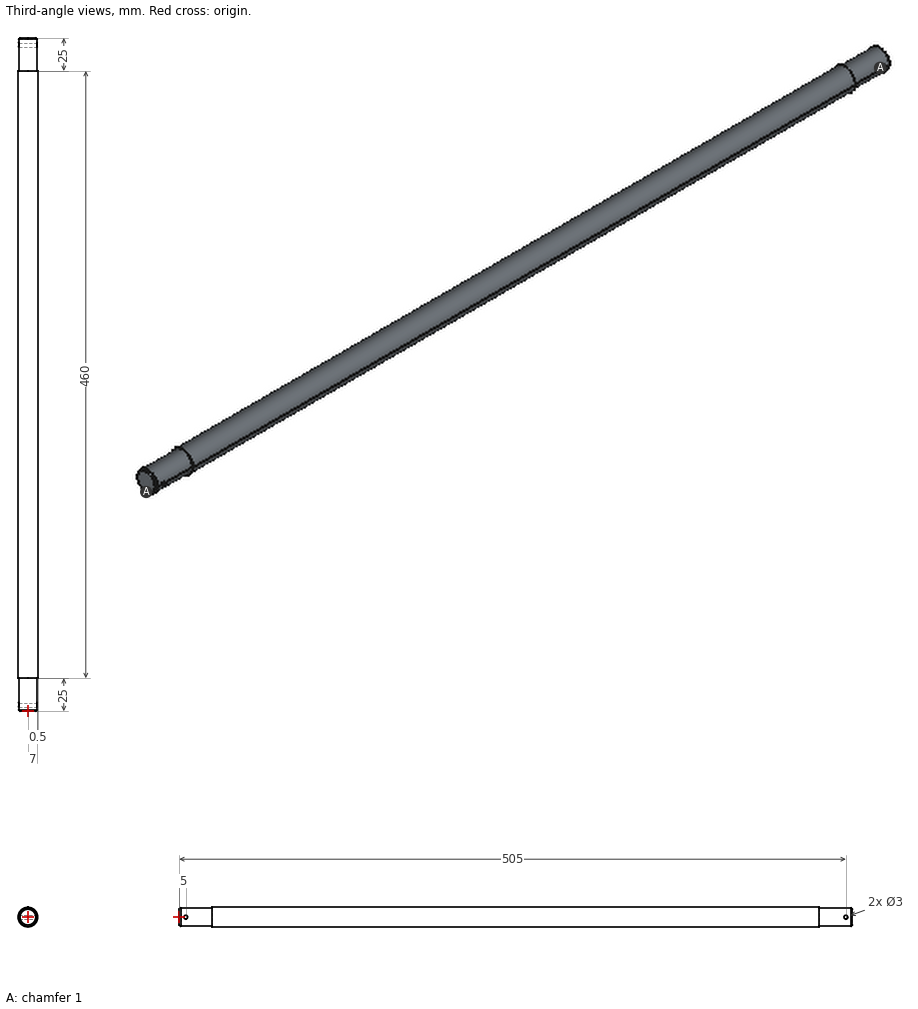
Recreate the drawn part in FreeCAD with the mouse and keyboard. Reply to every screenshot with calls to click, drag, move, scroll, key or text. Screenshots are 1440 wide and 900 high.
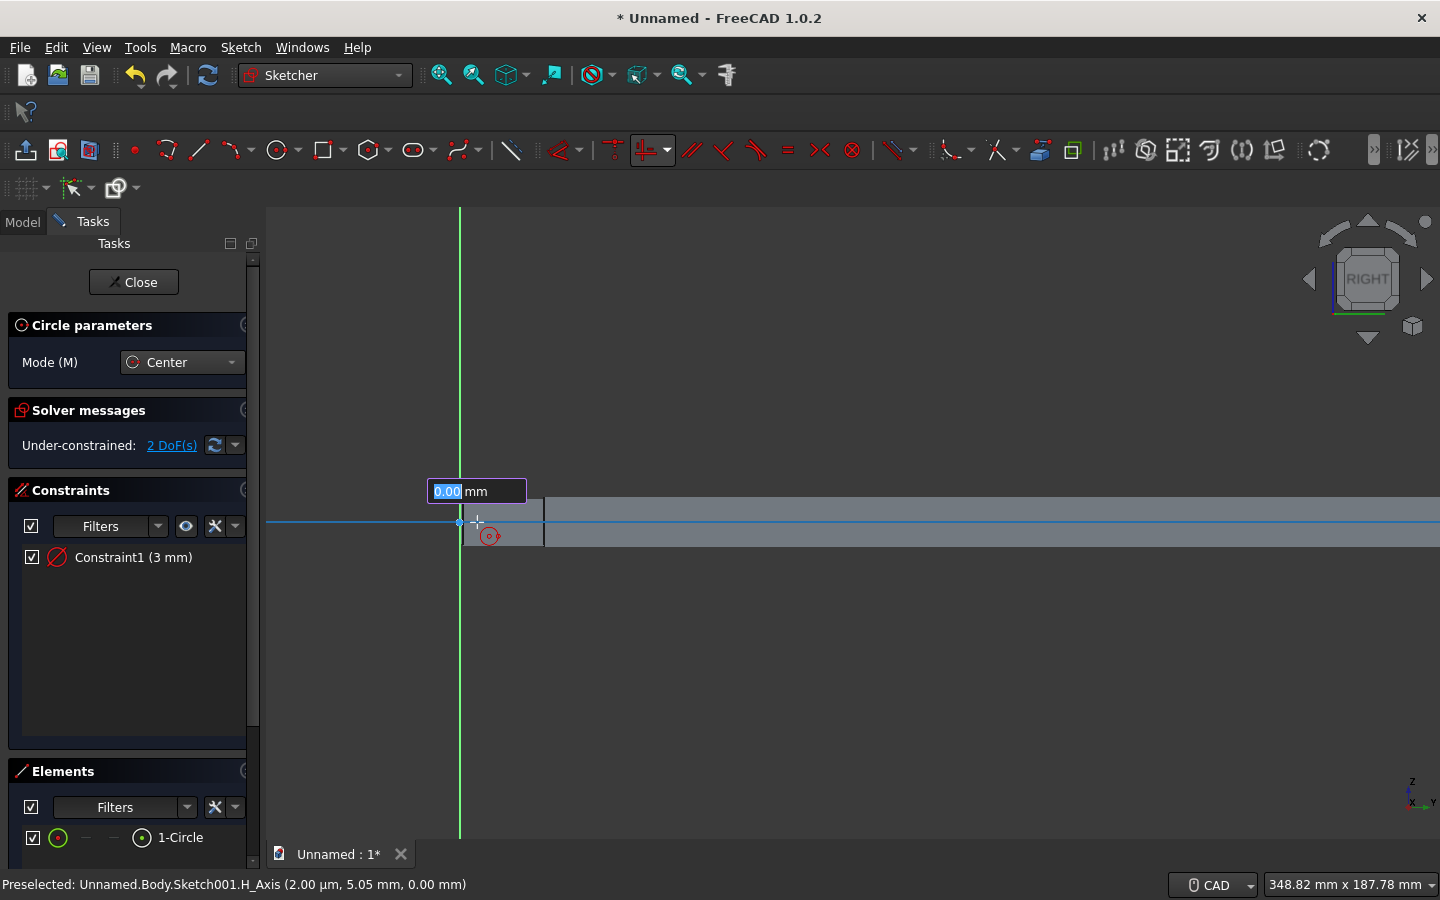
scroll(475, 527, up, 7)
move(475, 525)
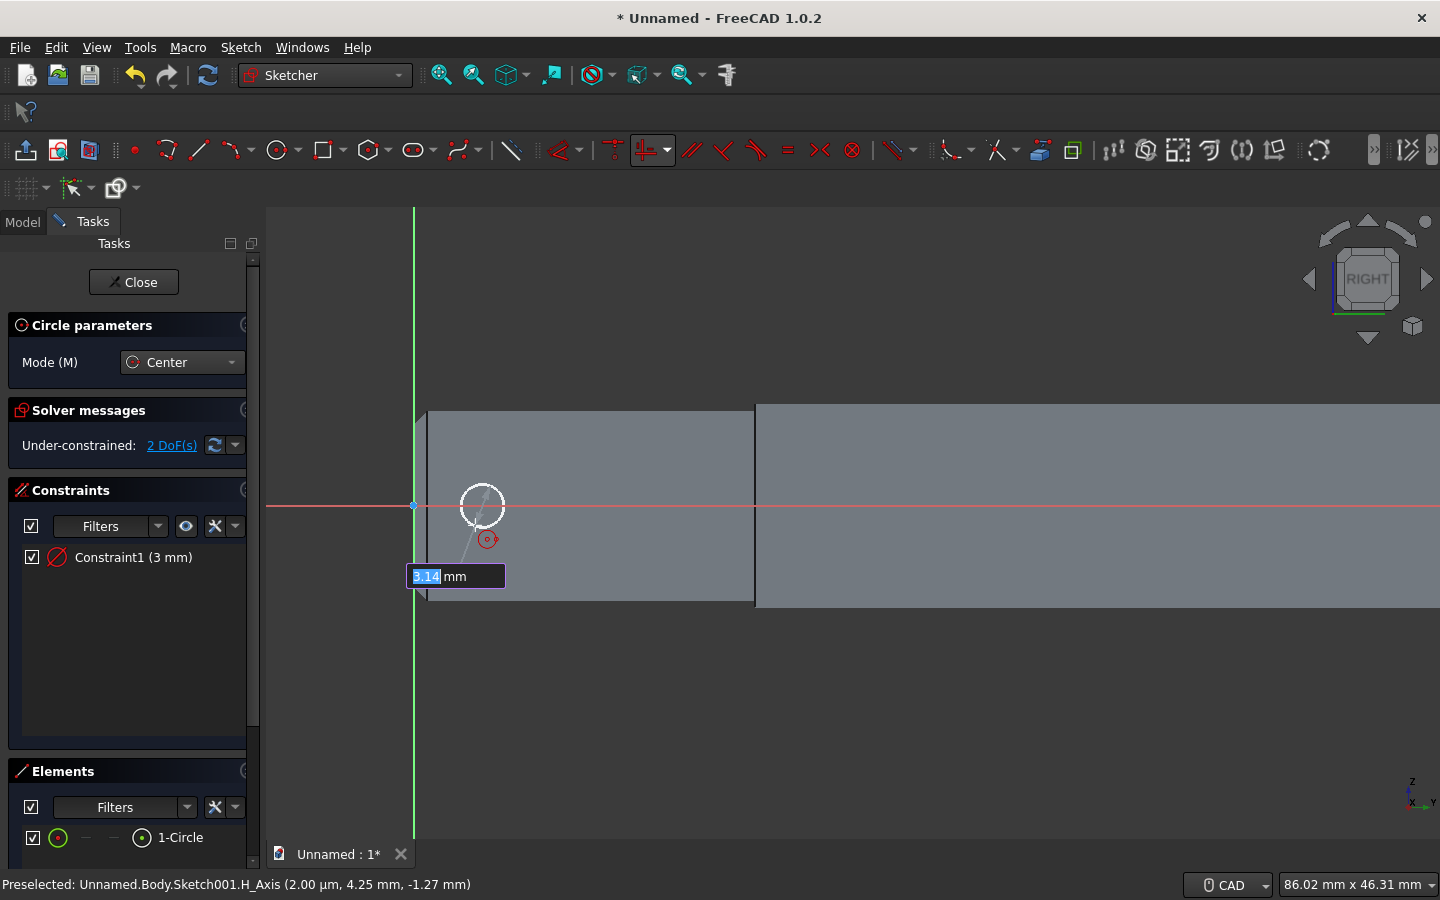
text(3)
key(Return)
key(Escape)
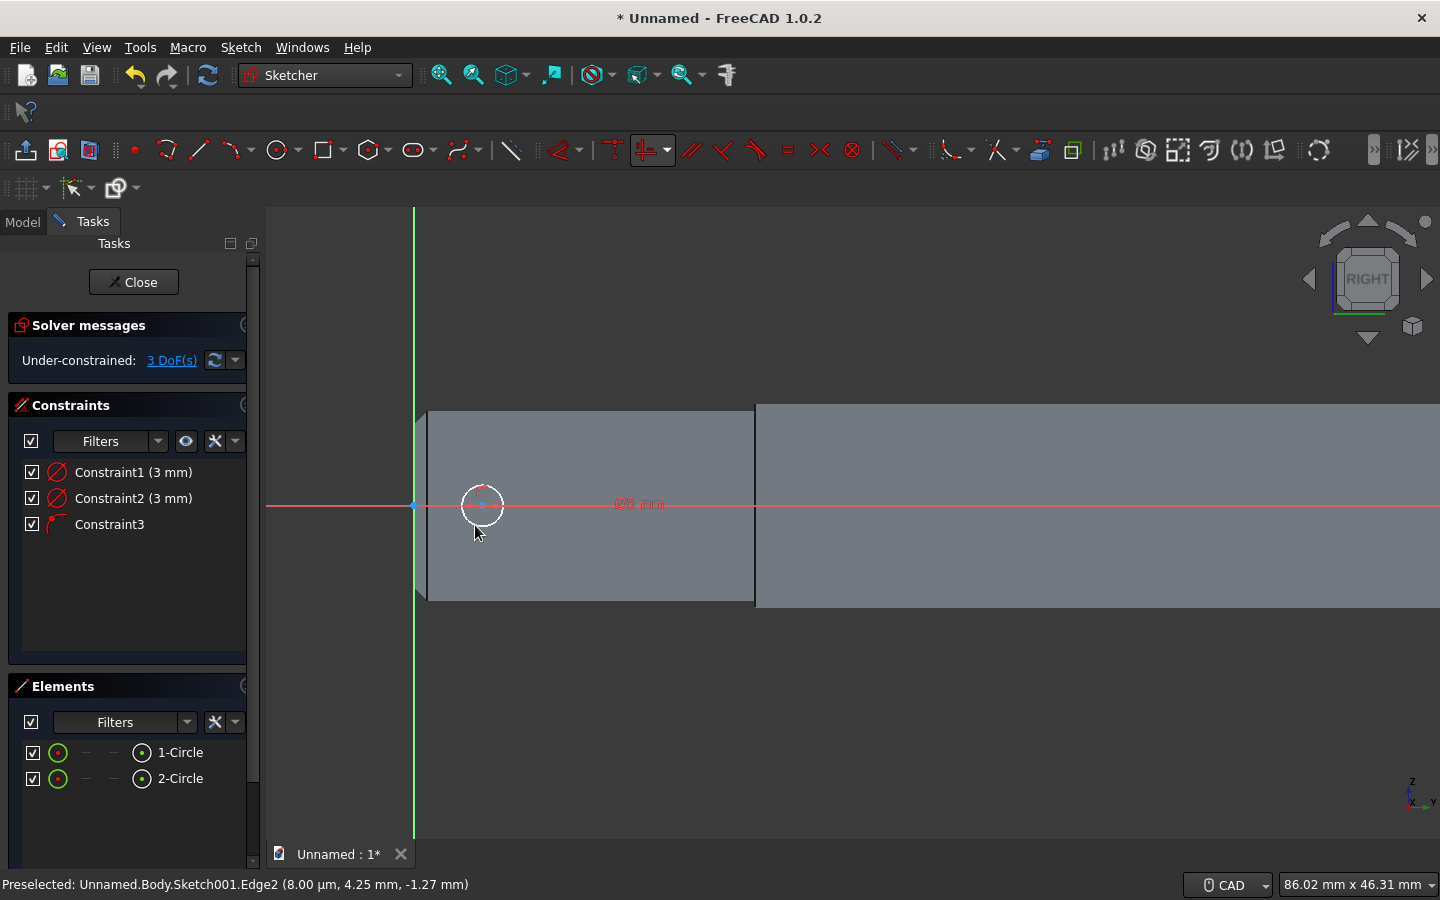
scroll(477, 525, down, 12)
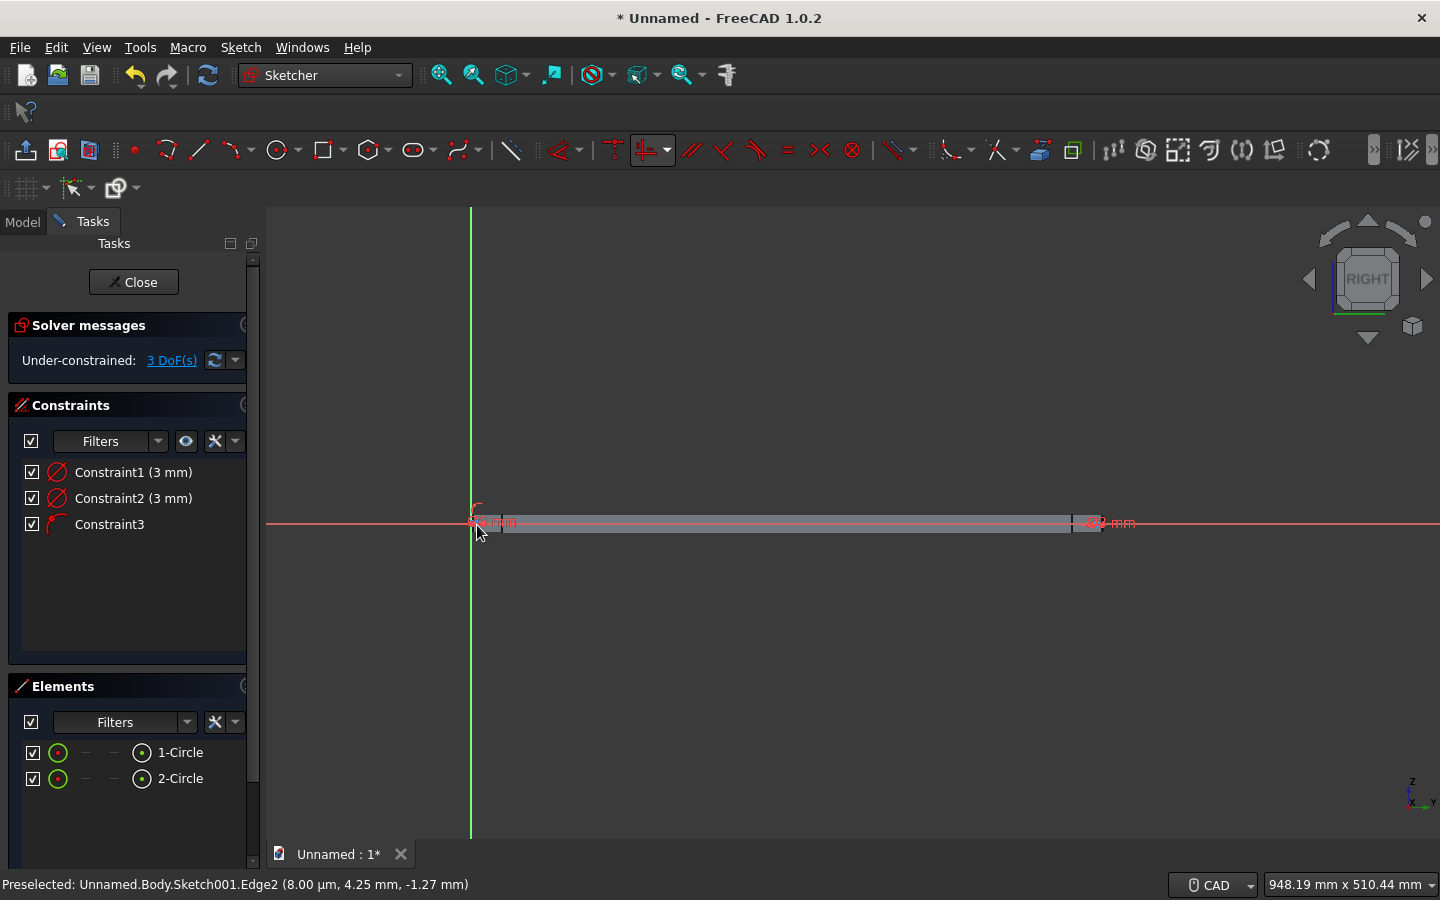
click(1097, 525)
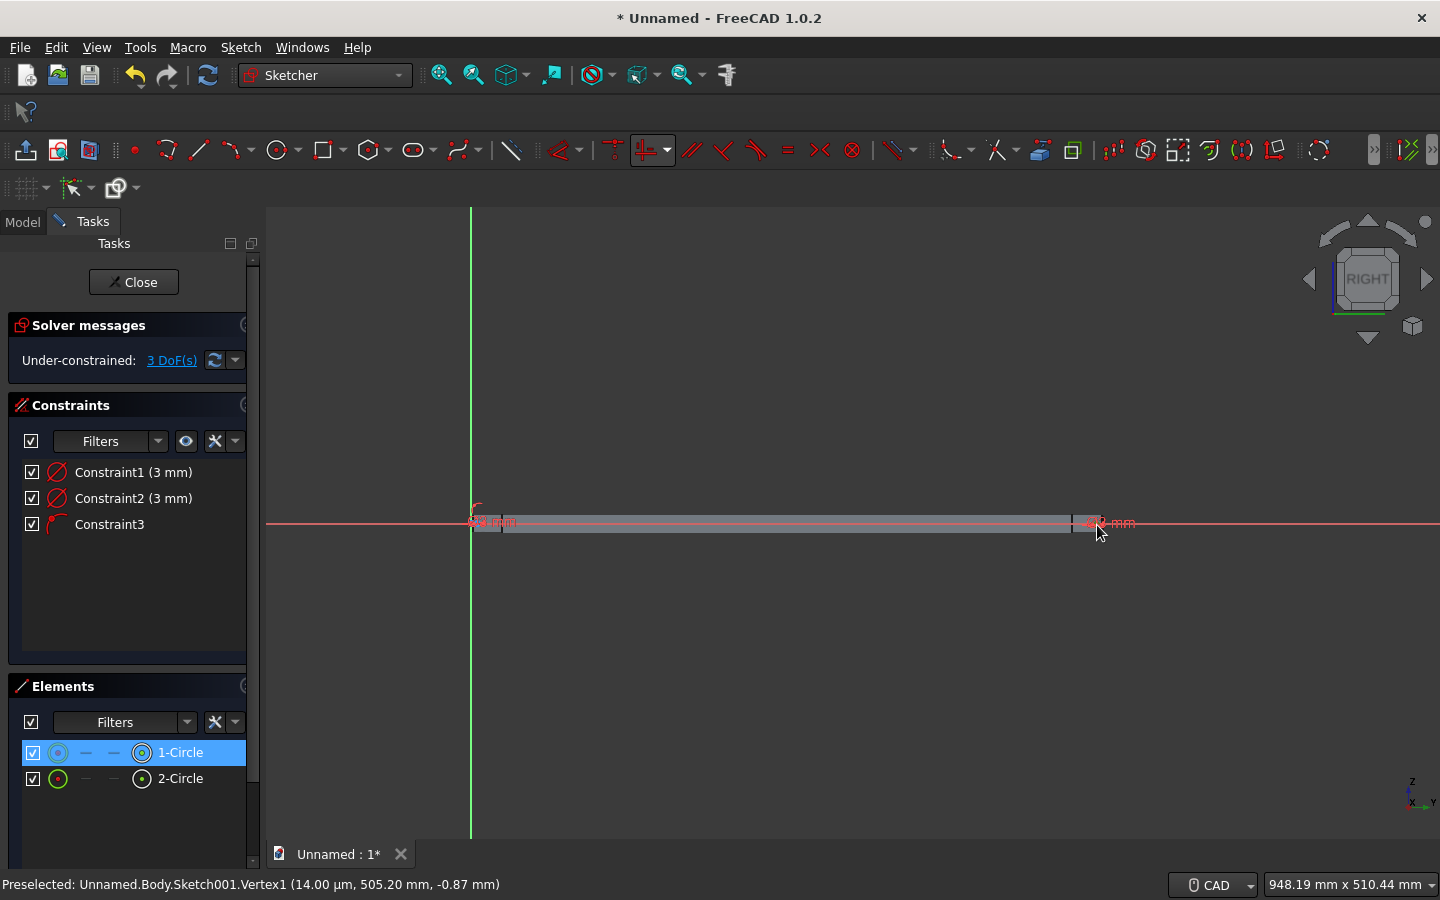
click(364, 524)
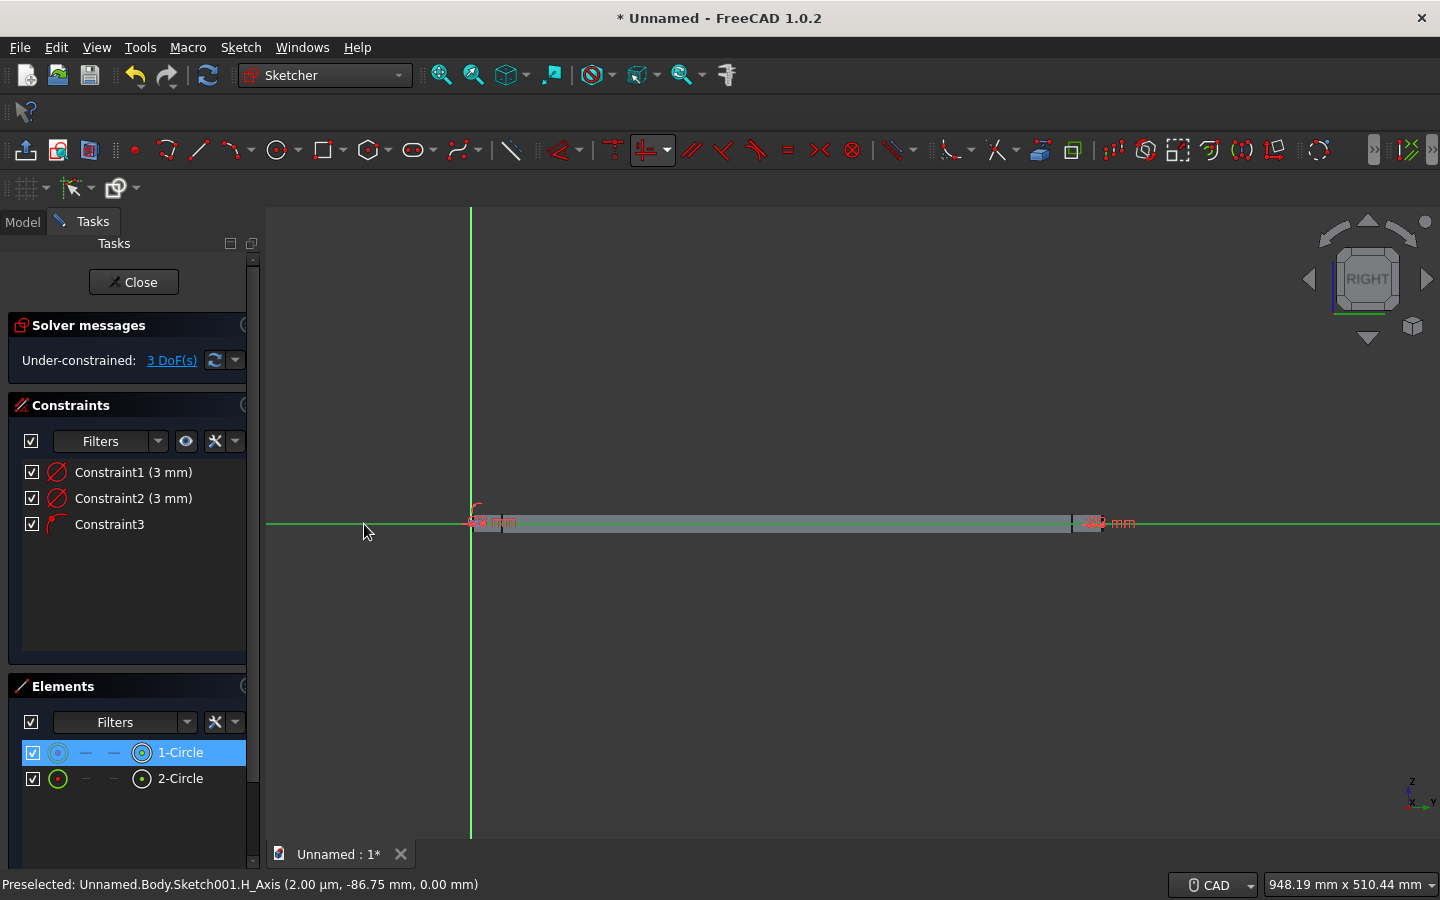
click(614, 150)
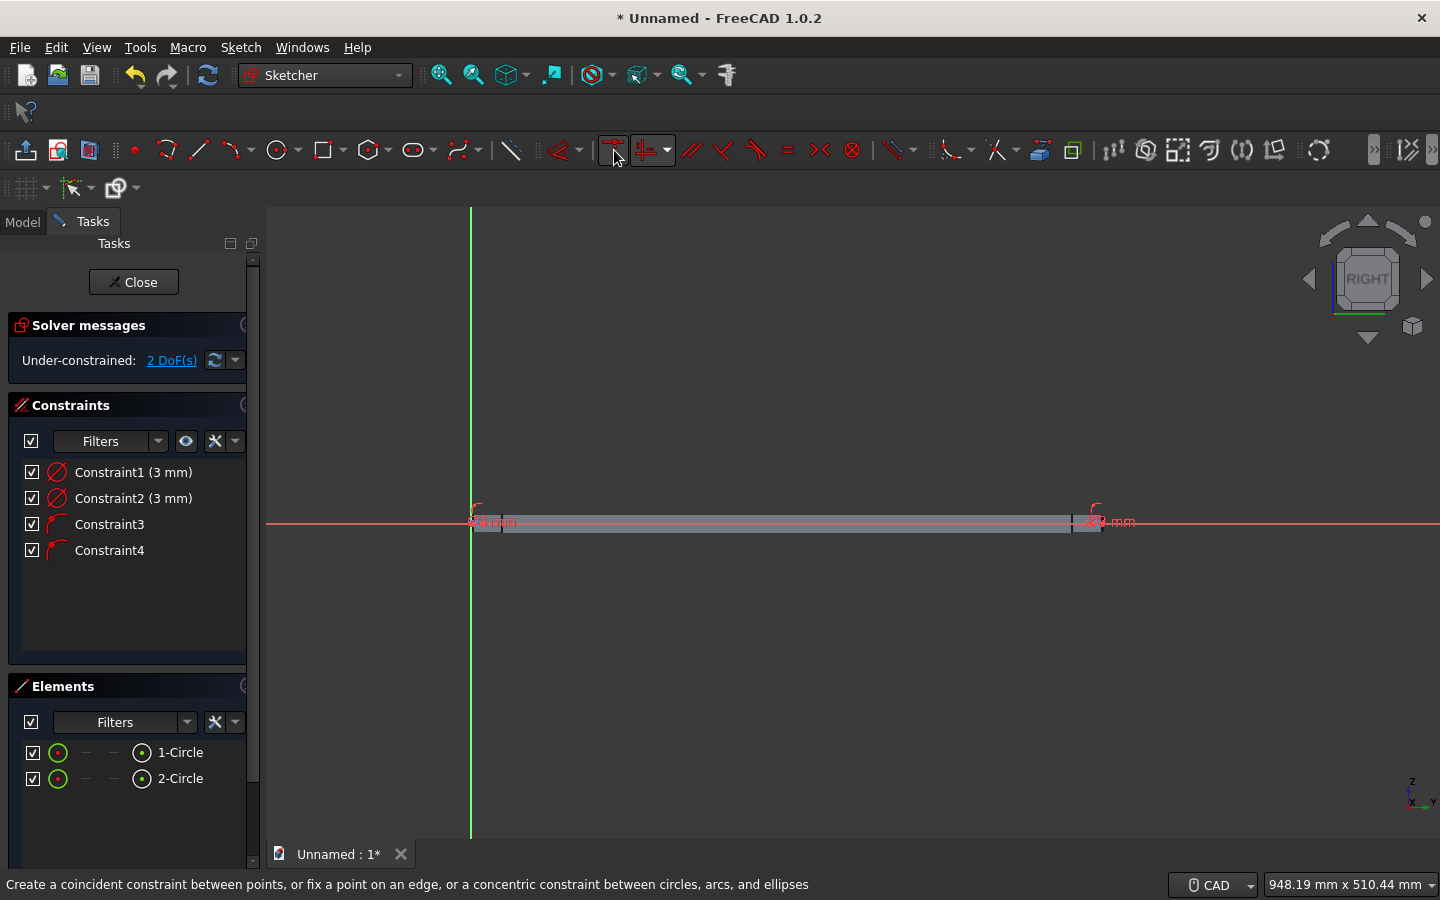
click(558, 150)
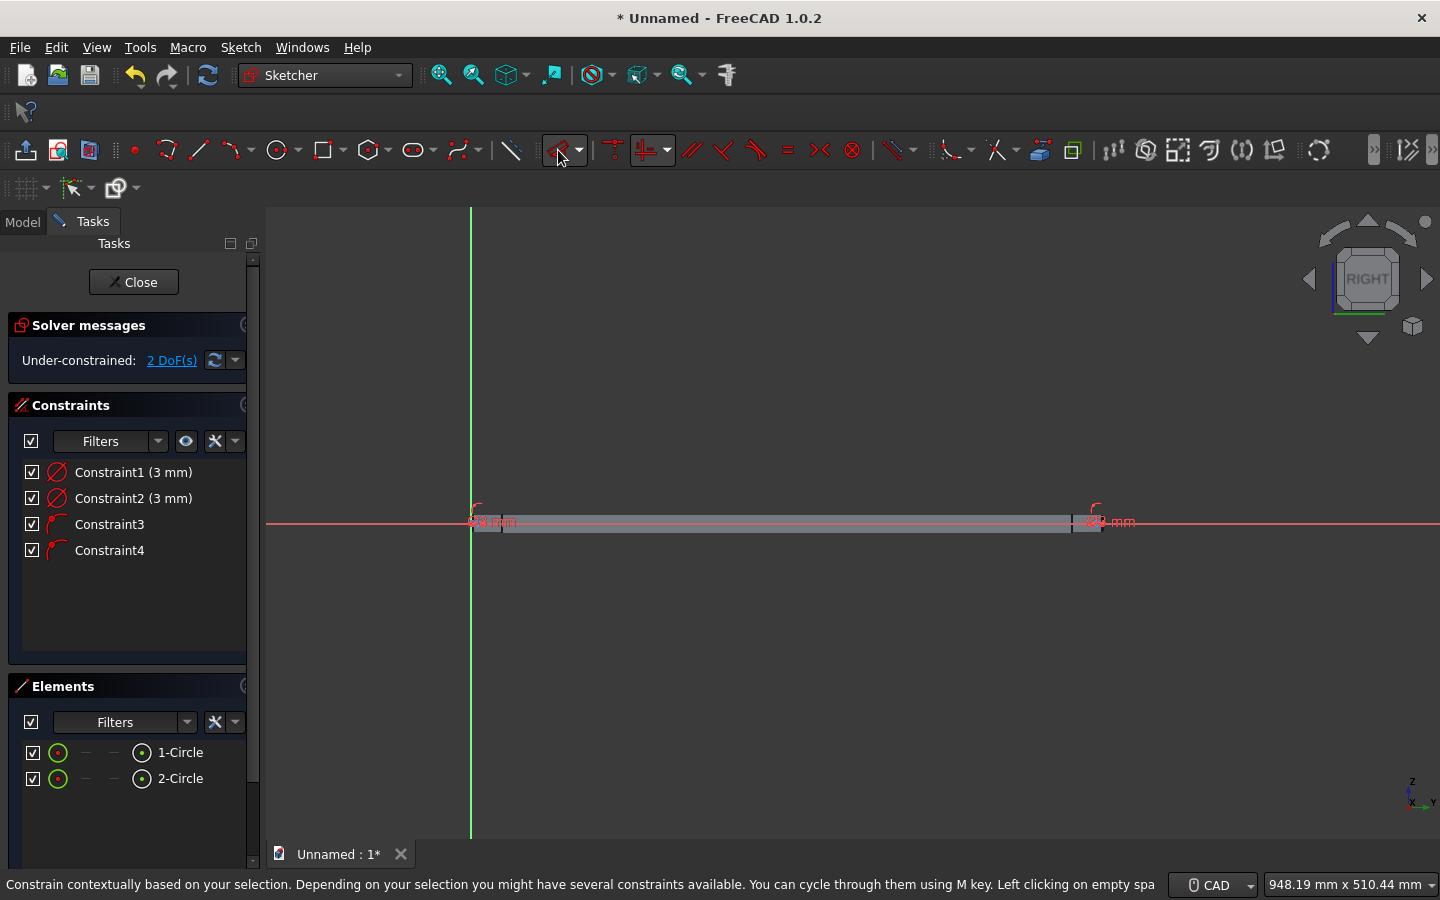
scroll(478, 524, up, 10)